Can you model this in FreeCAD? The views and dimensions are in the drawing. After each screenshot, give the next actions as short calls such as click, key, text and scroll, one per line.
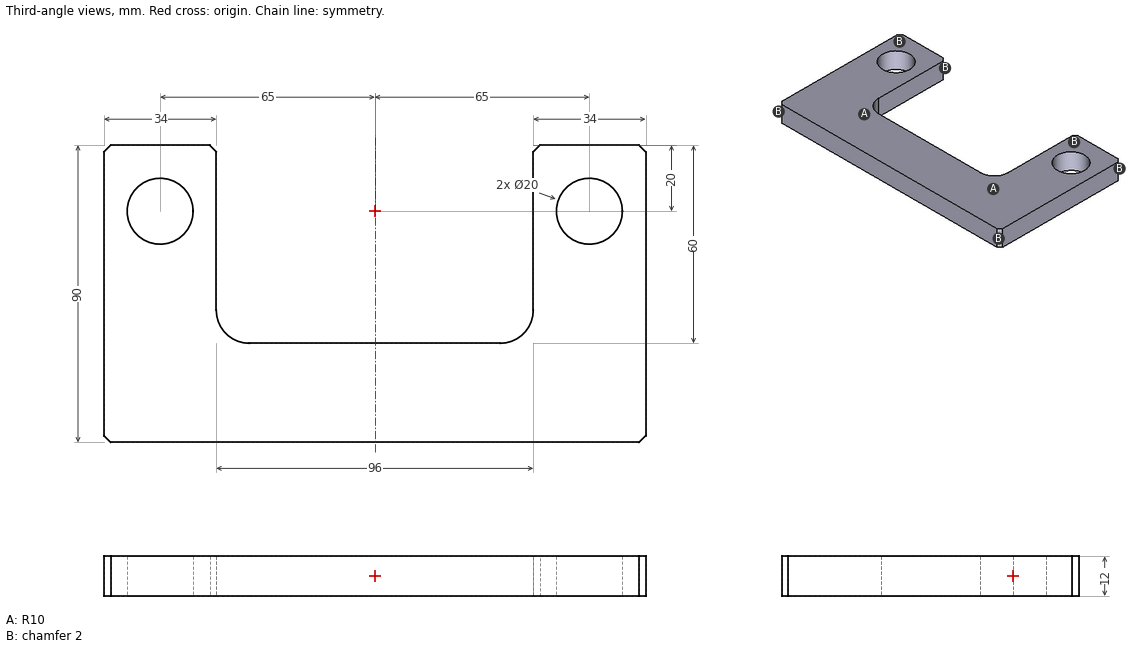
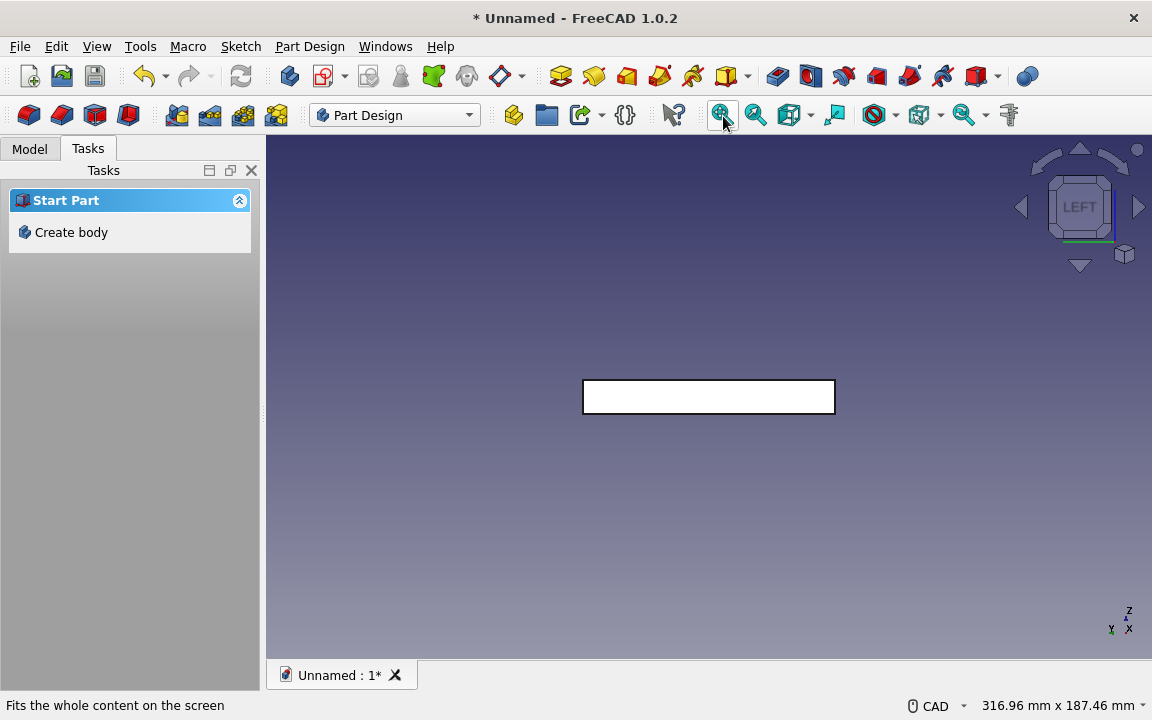
key(v)
key(3)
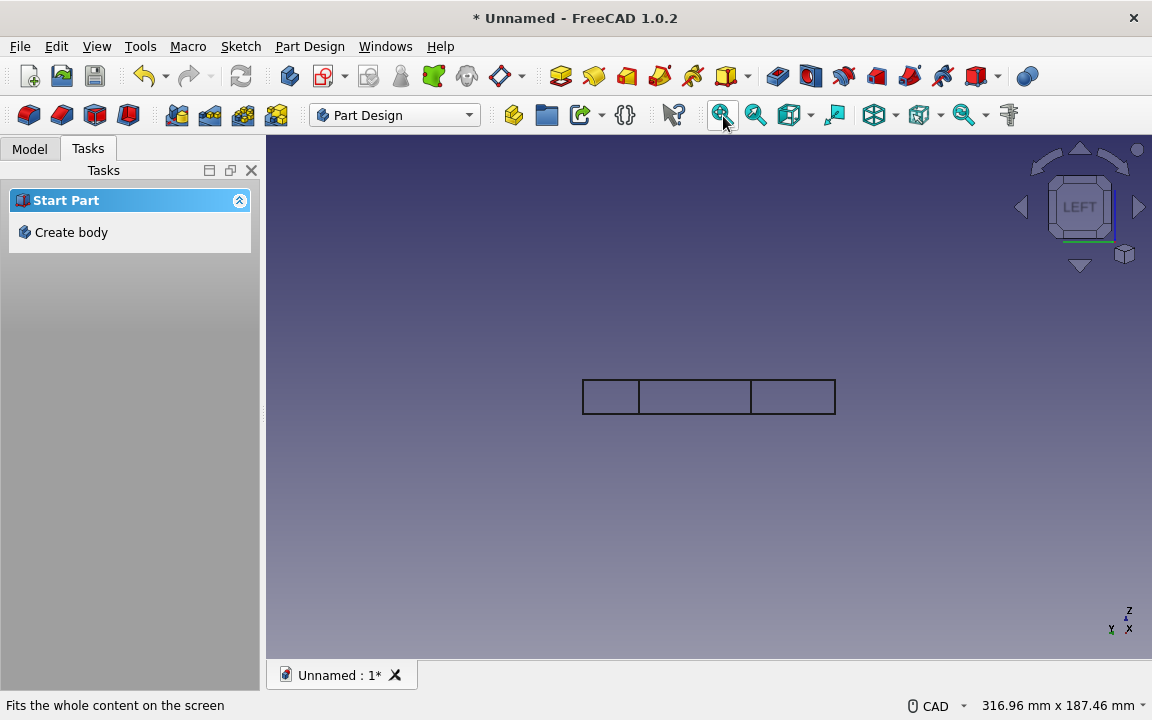
key(0)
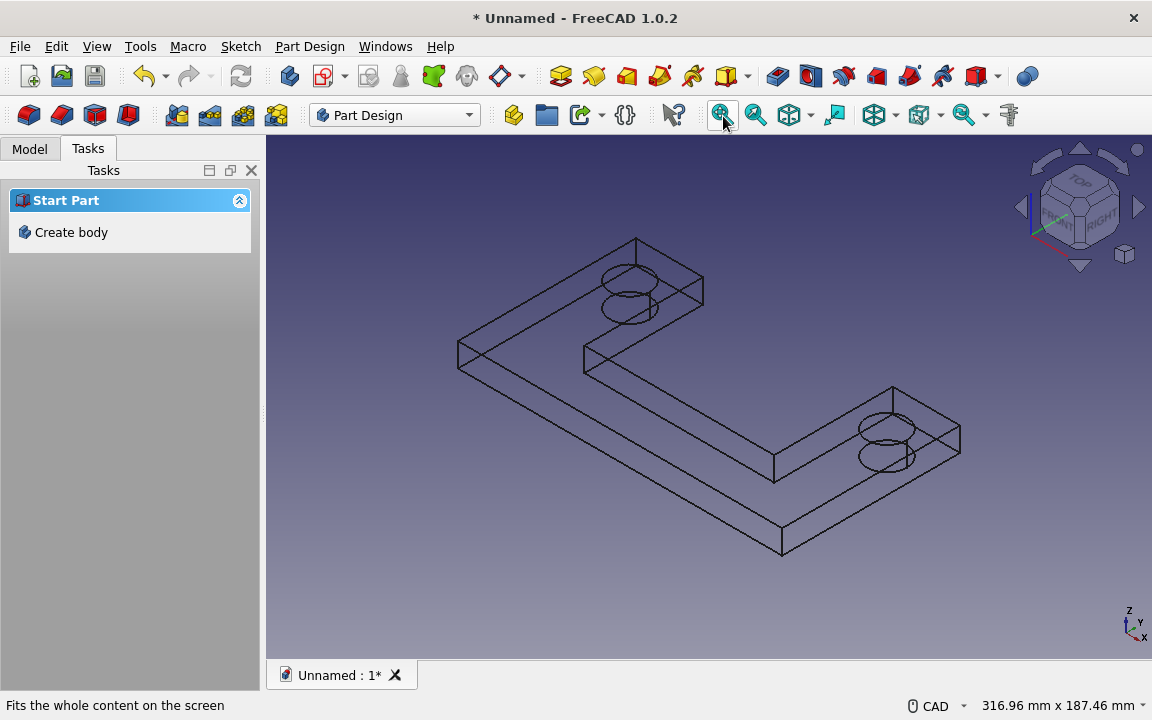
click(584, 358)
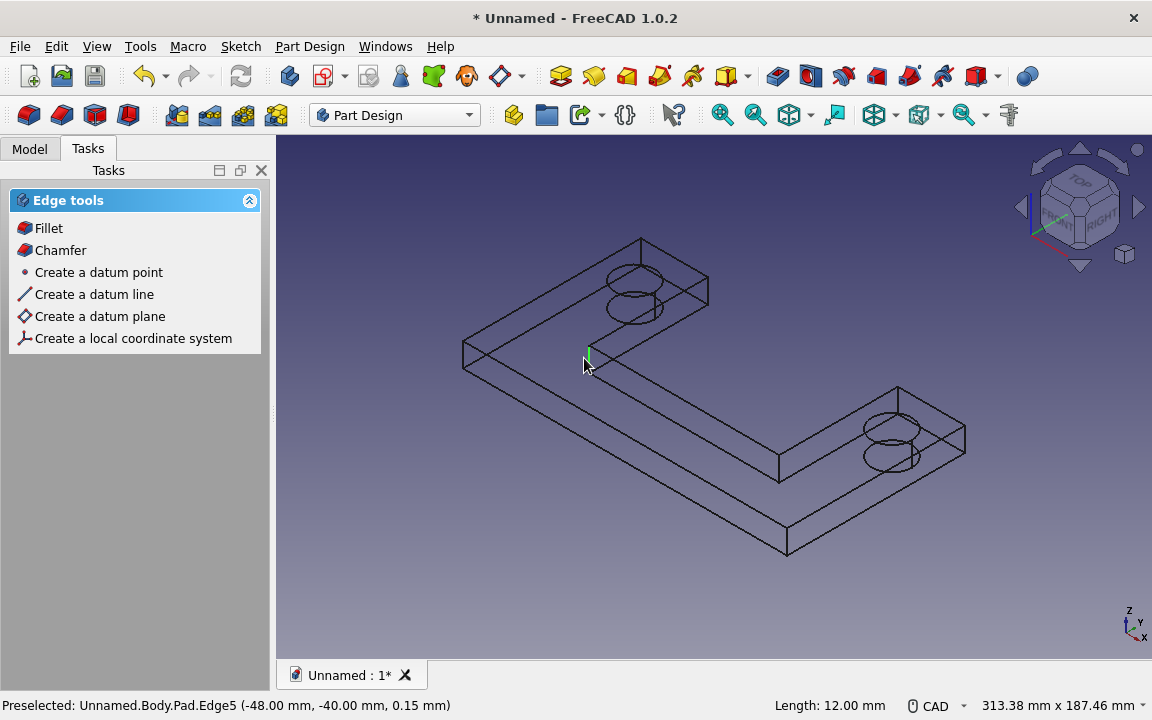
click(779, 468, ctrl)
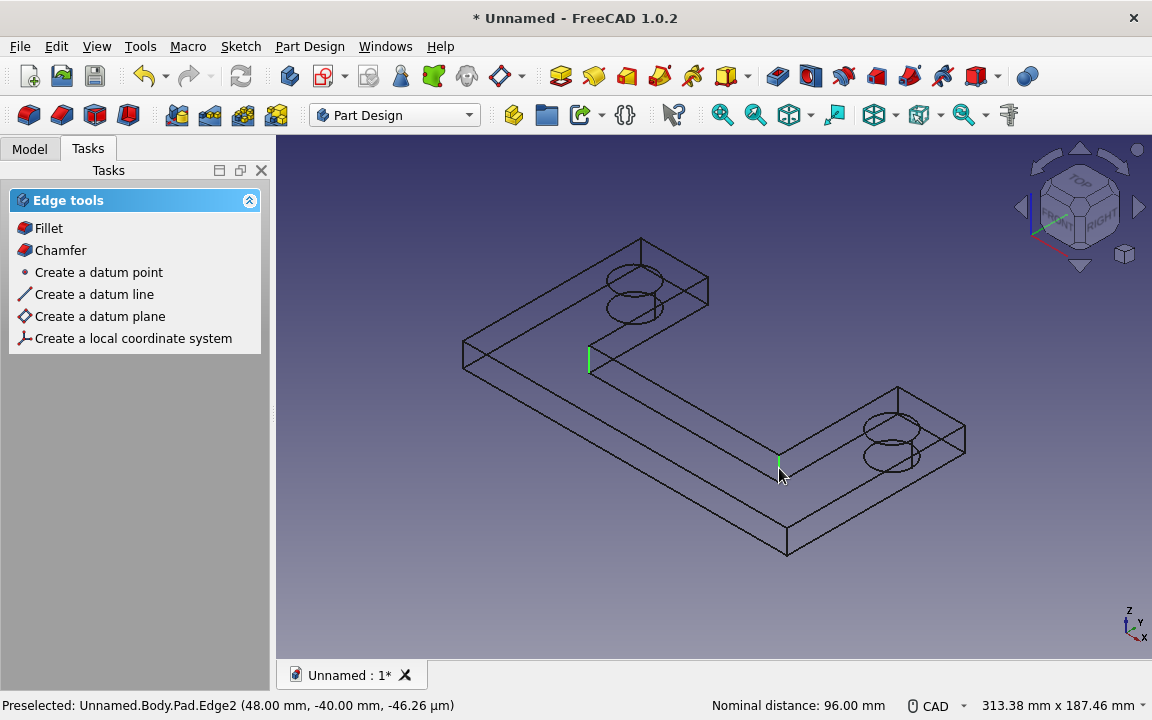
key(v)
key(1)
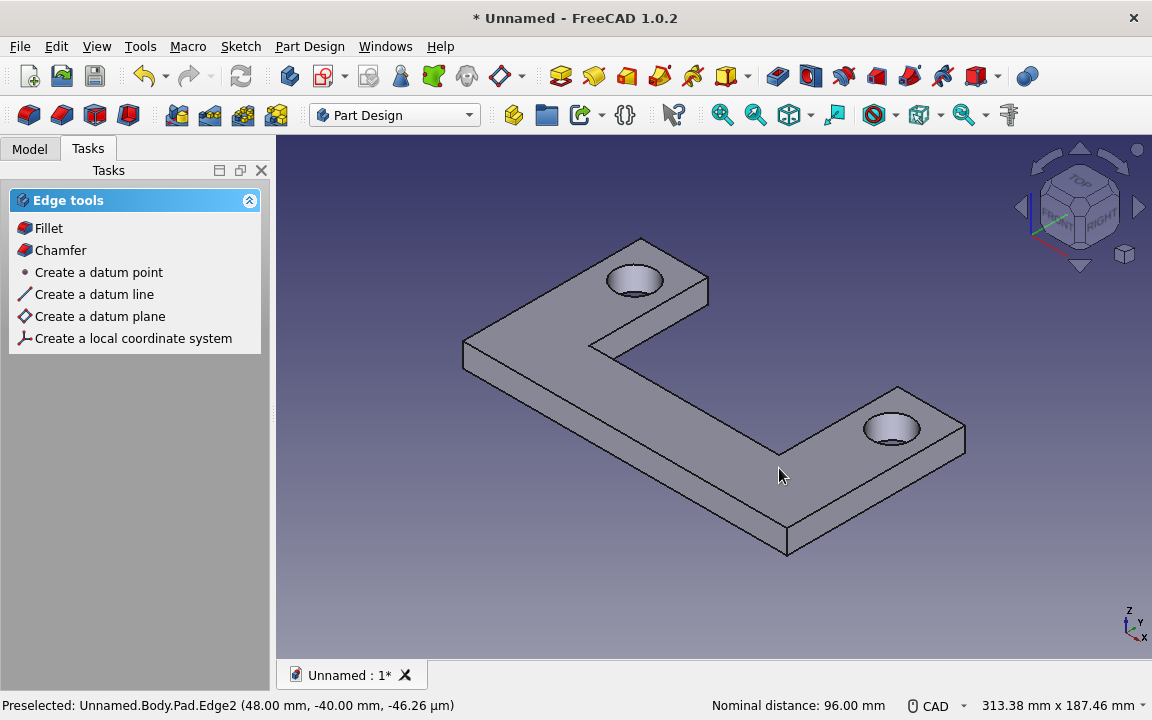
click(29, 116)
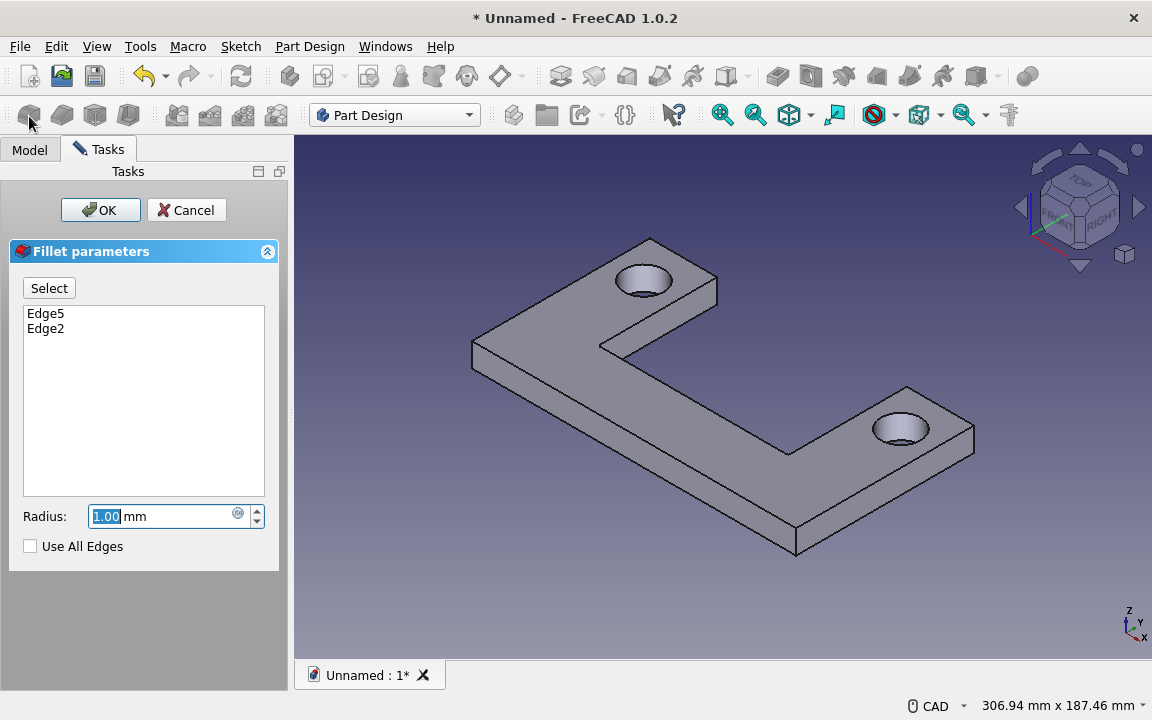
text(10)
key(Tab)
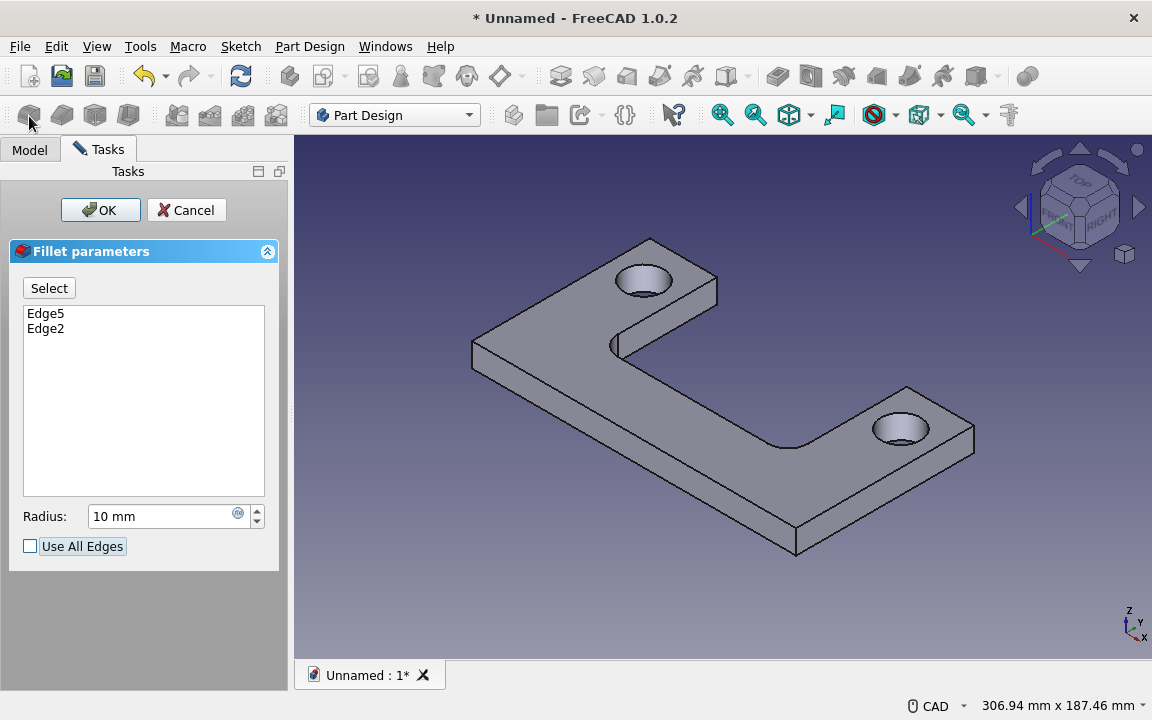
click(101, 210)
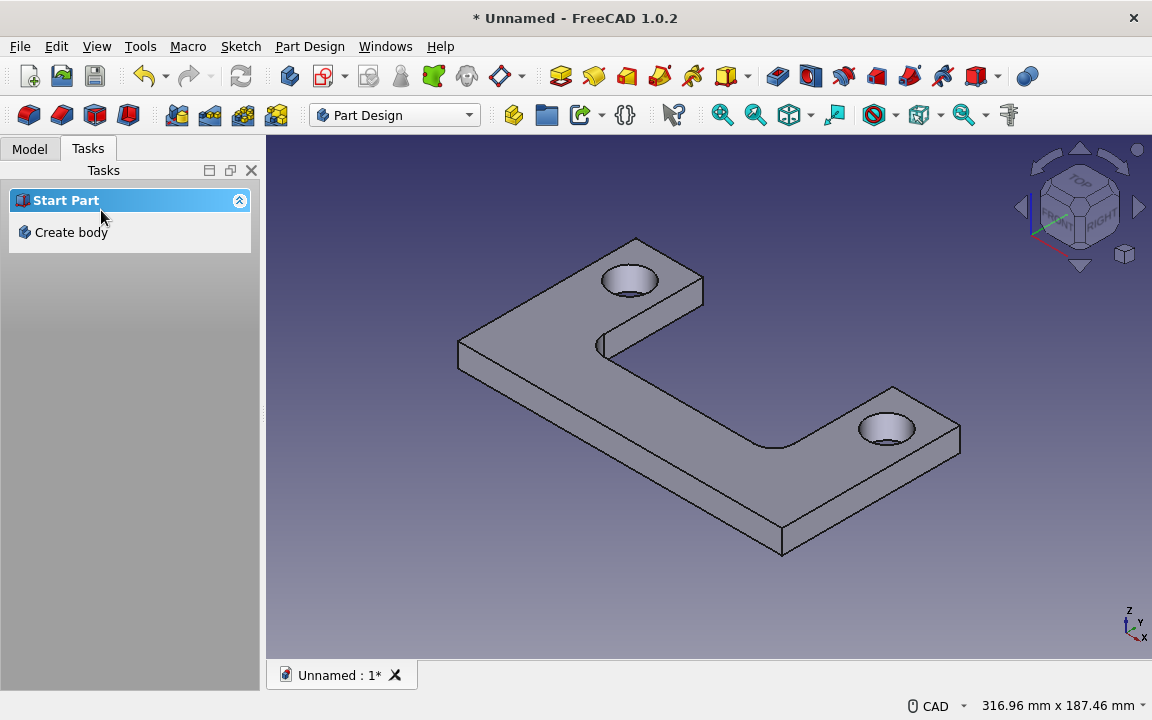
click(782, 541)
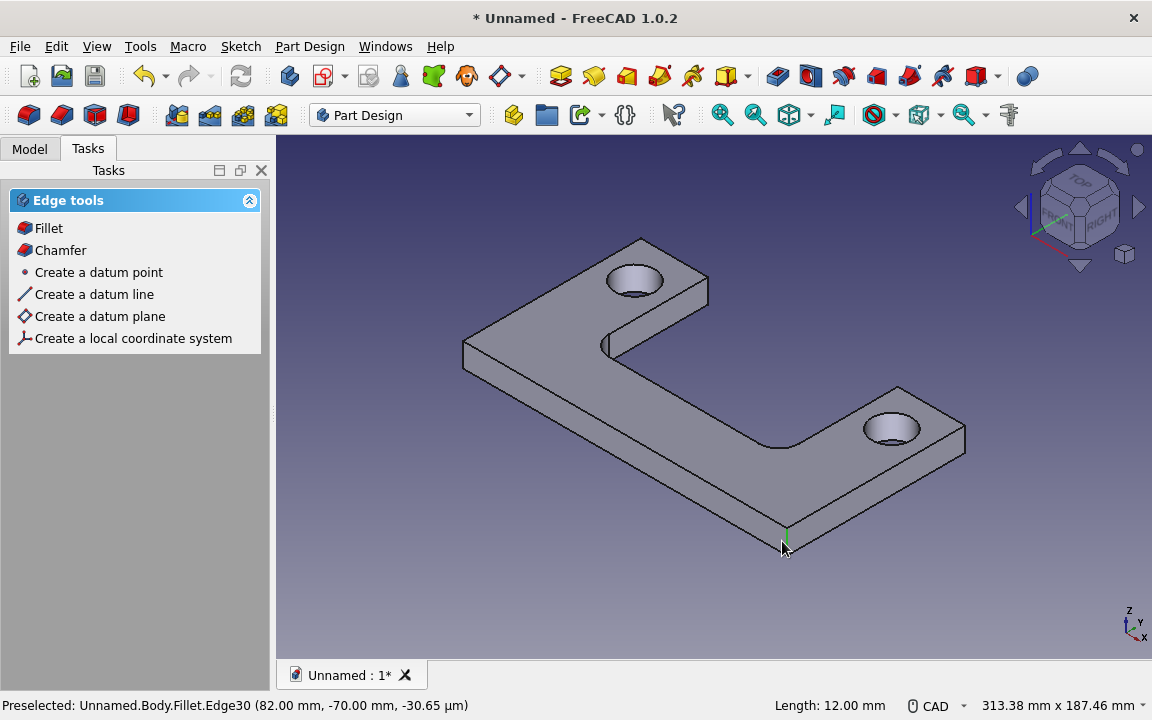
key(2)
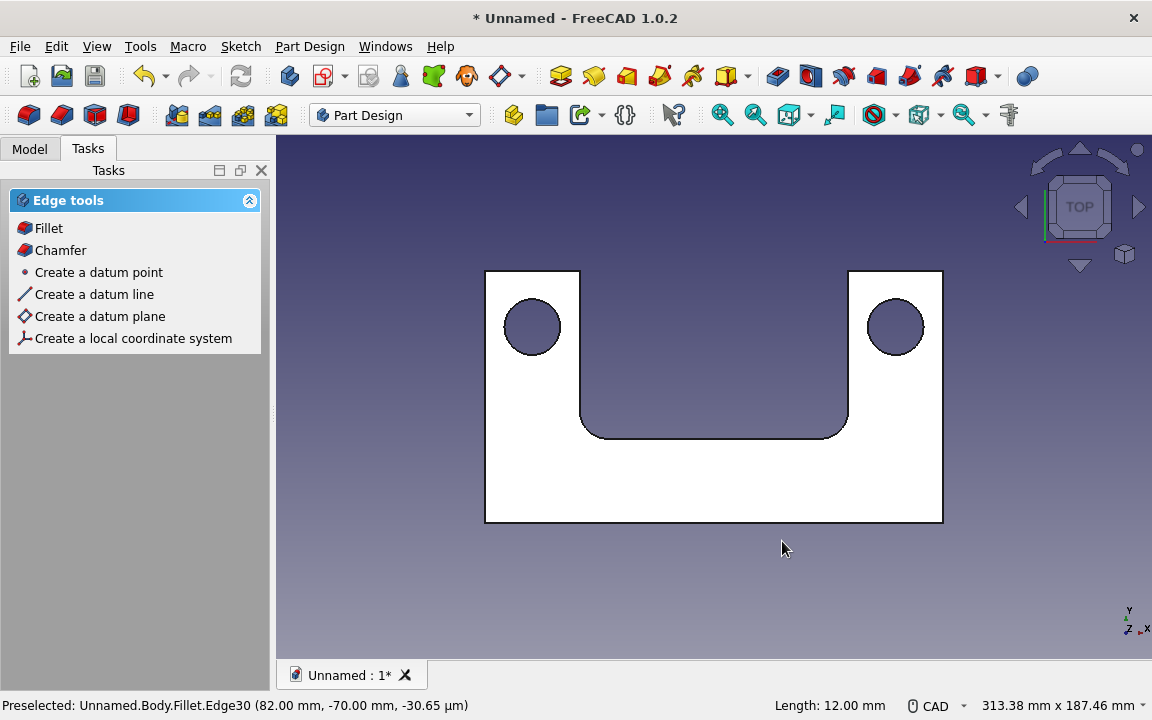
key(0)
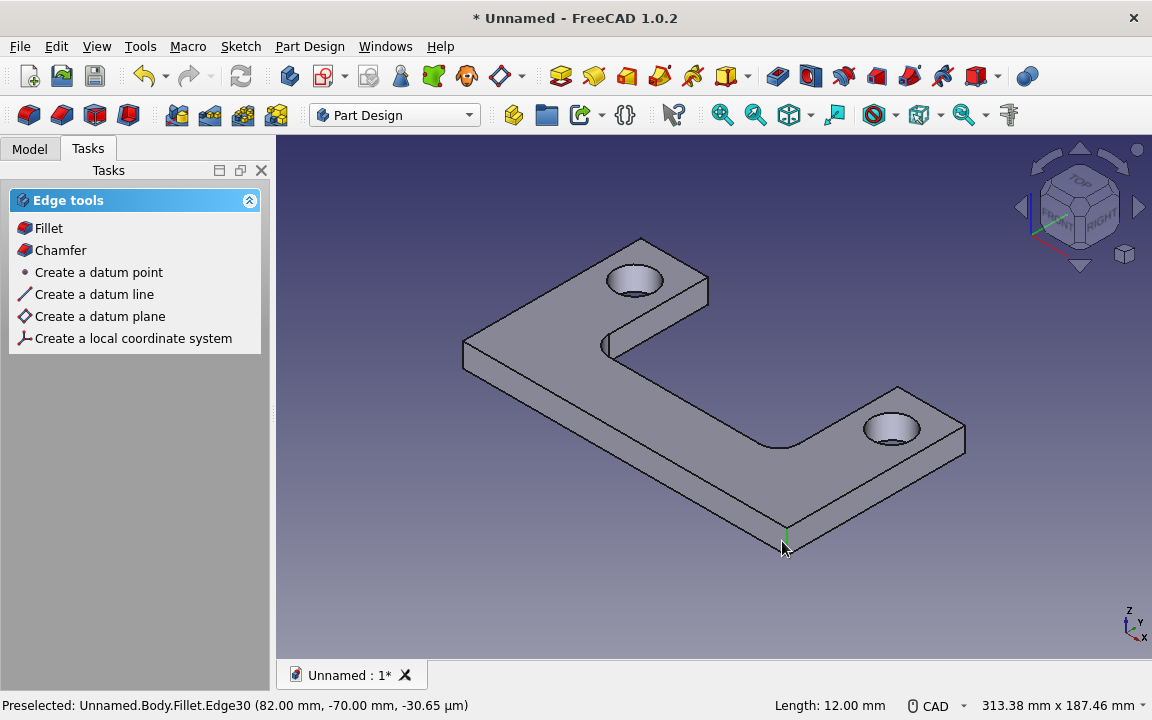
key(1)